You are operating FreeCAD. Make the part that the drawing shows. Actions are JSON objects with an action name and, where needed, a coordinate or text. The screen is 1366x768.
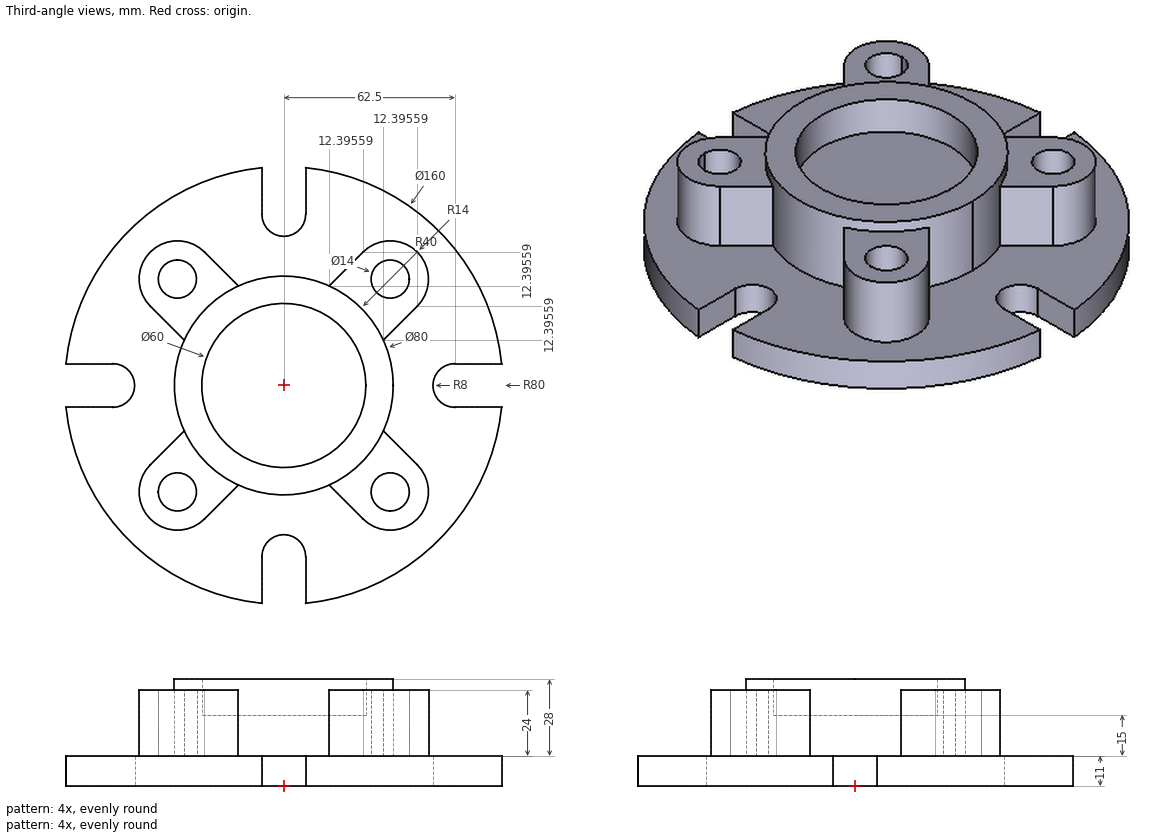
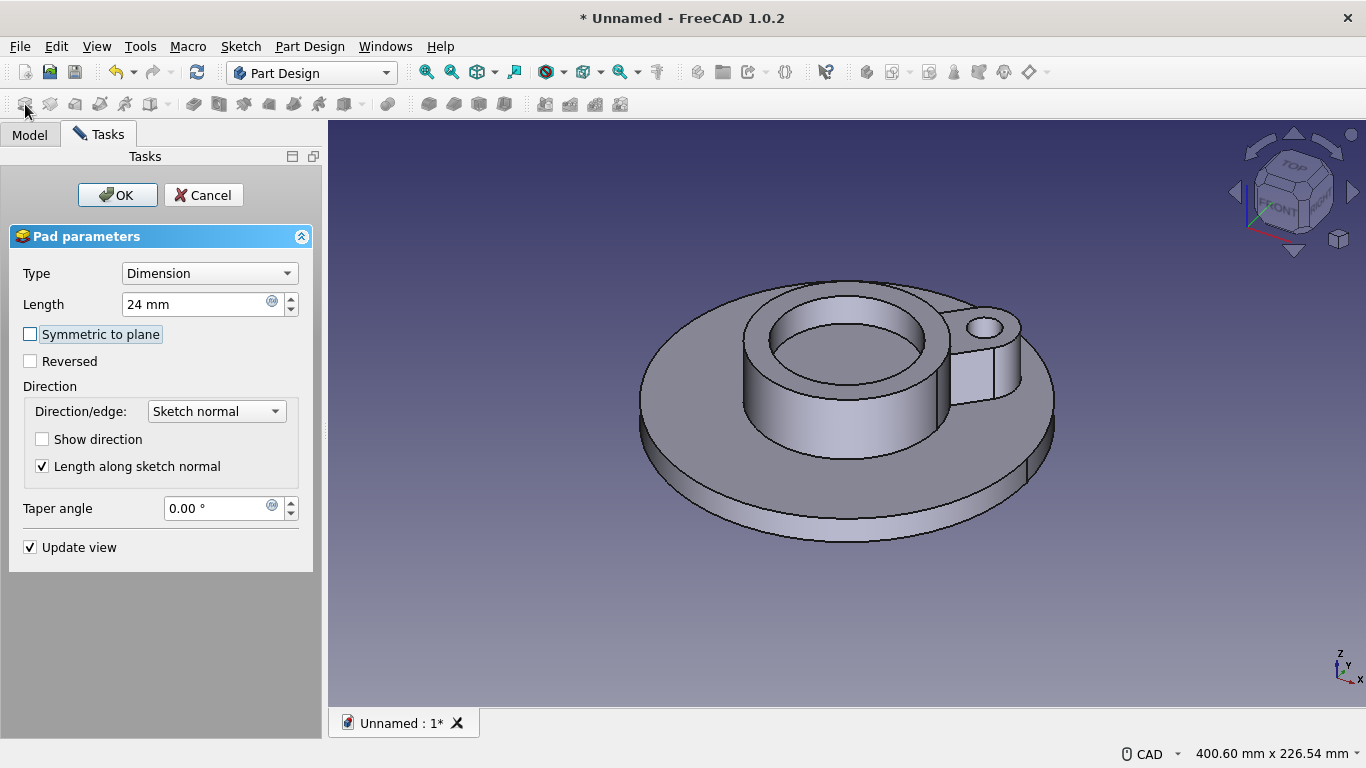
{"action": "left_click", "coordinate": [118, 195]}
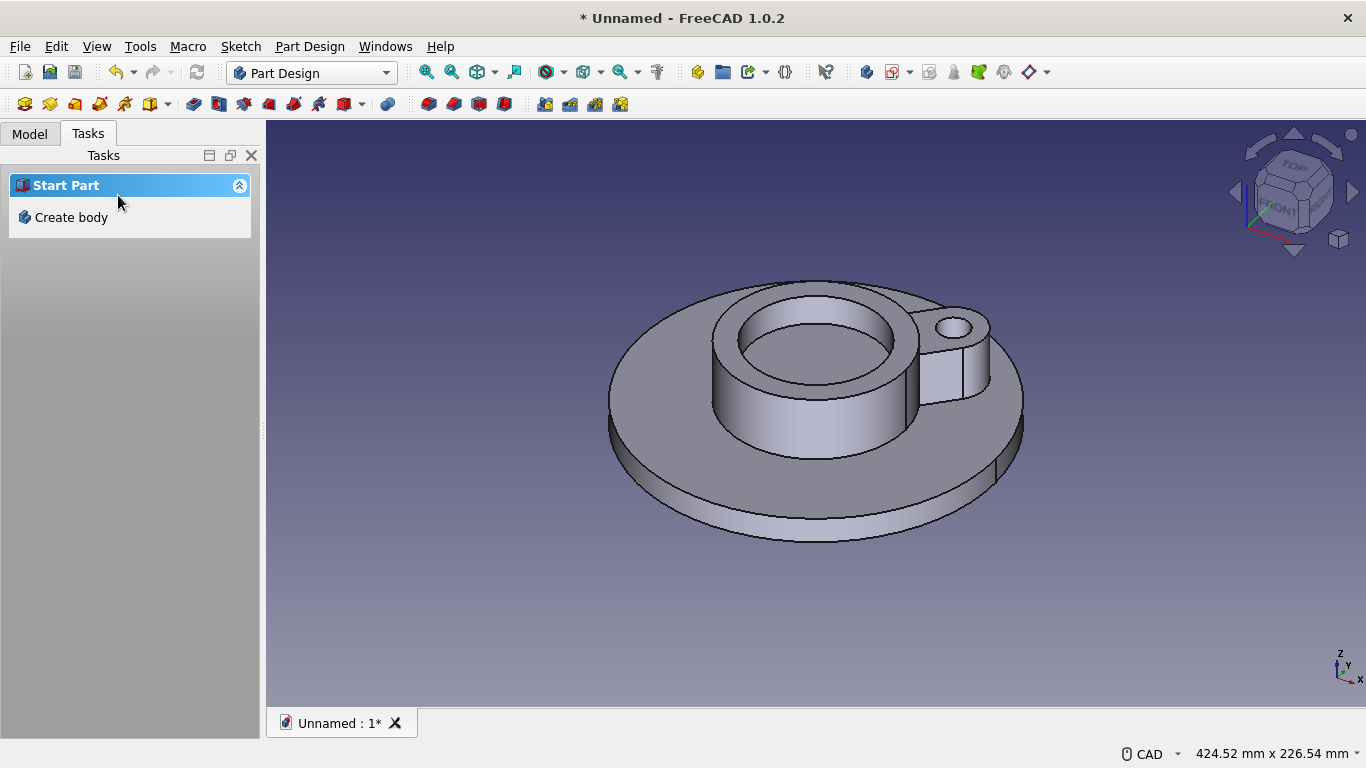
{"action": "left_click", "coordinate": [30, 134]}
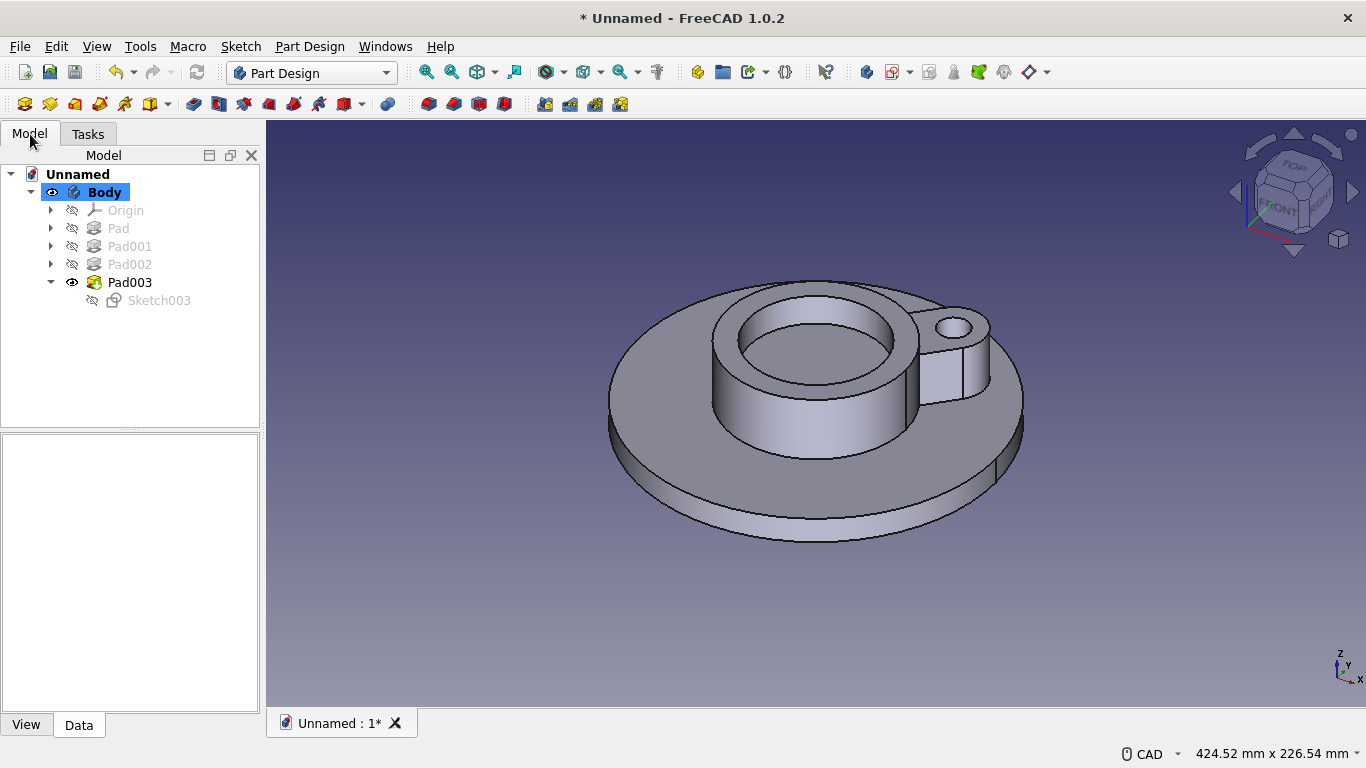
{"action": "left_click", "coordinate": [117, 282]}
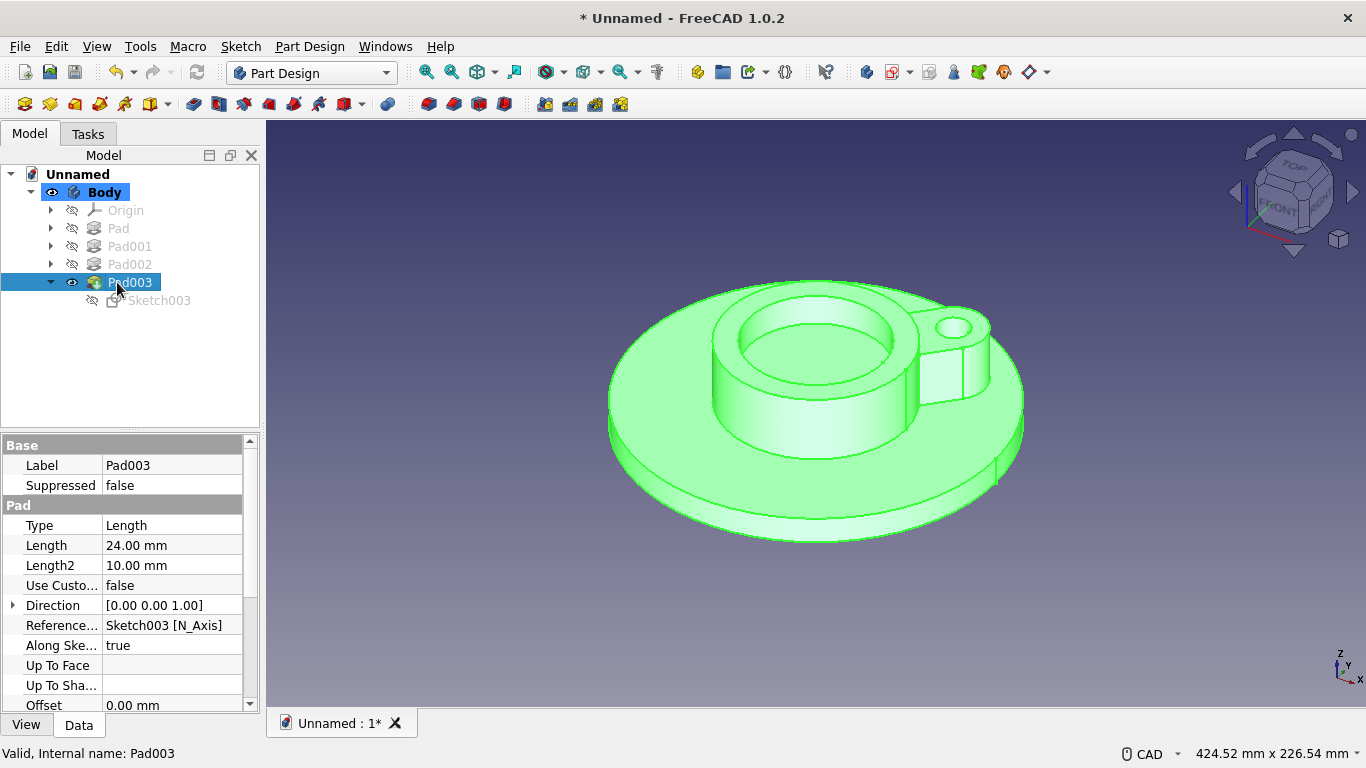
{"action": "left_click", "coordinate": [595, 104]}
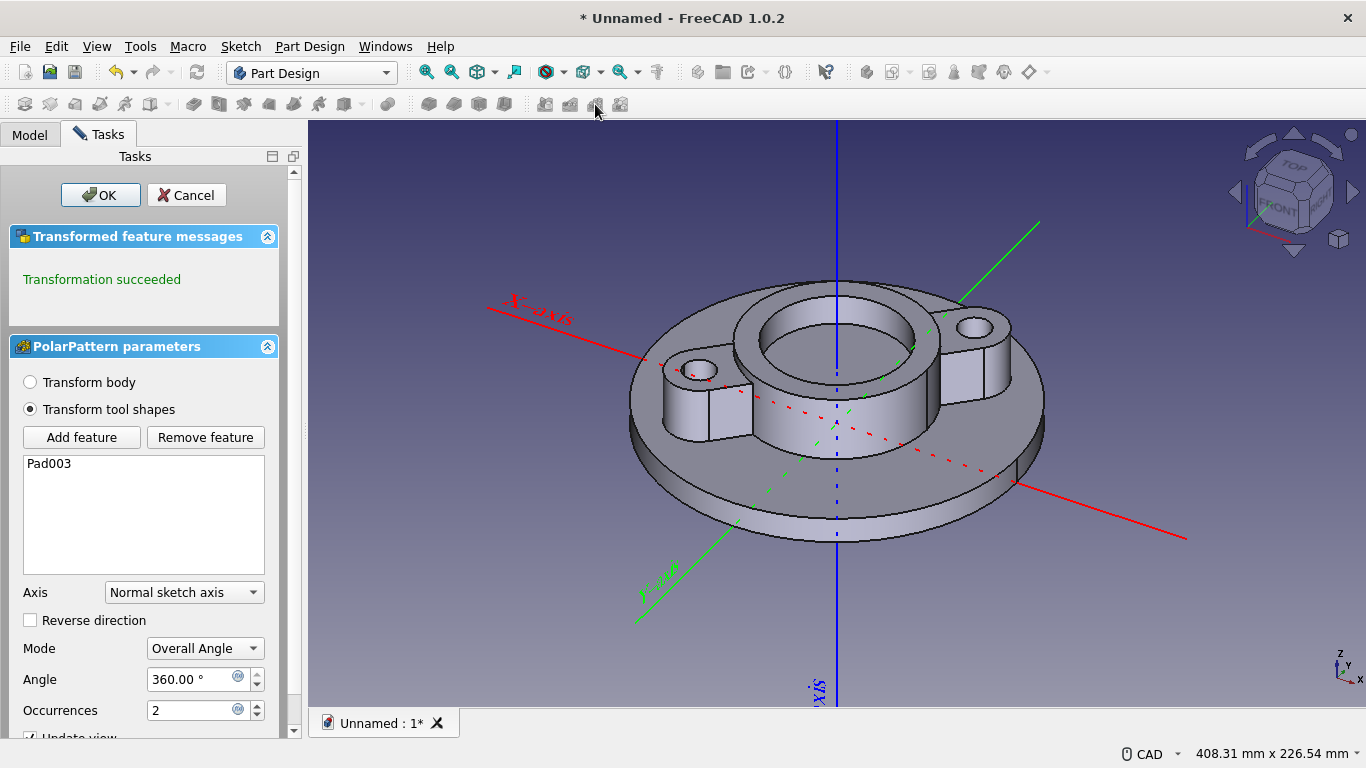
{"action": "left_click", "coordinate": [185, 592]}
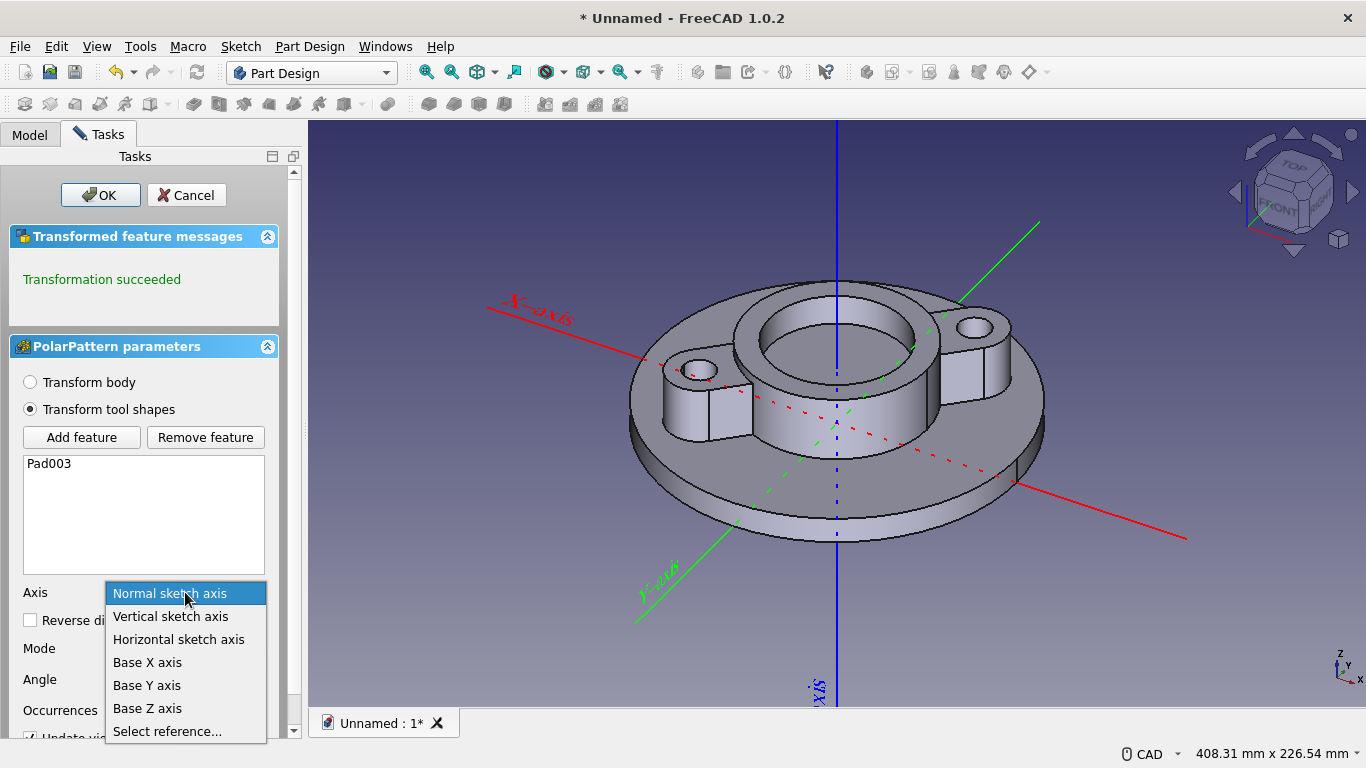
{"action": "left_click", "coordinate": [184, 708]}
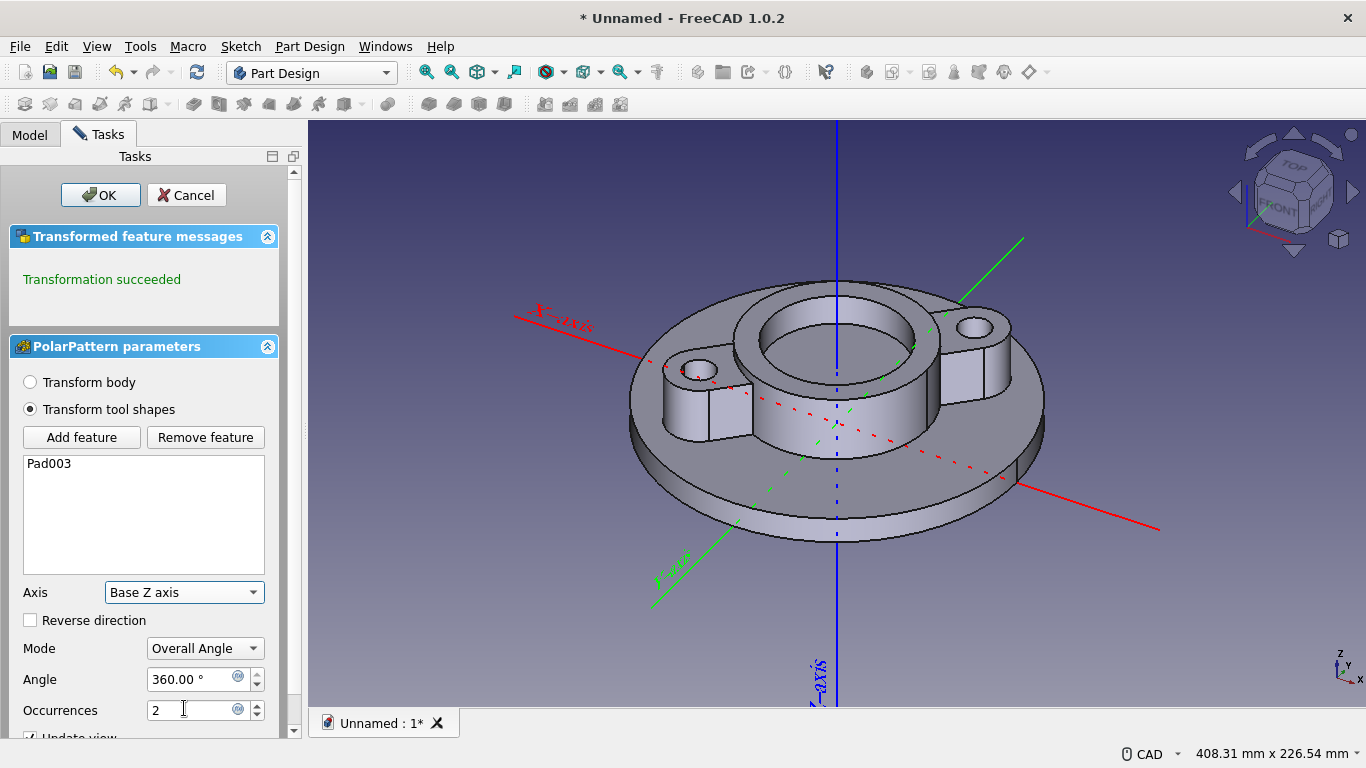
{"action": "triple_click", "coordinate": [199, 710]}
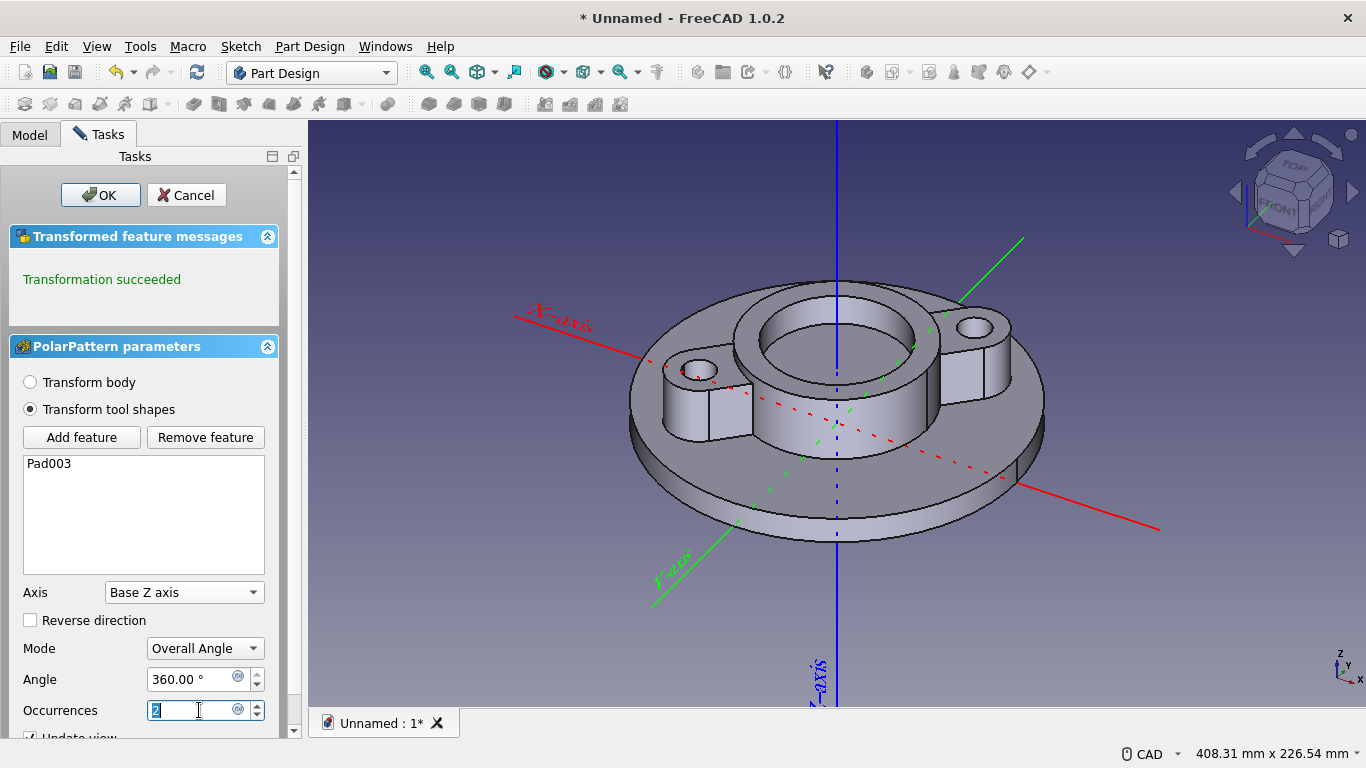
{"action": "type", "text": "4"}
{"action": "key", "text": "Tab"}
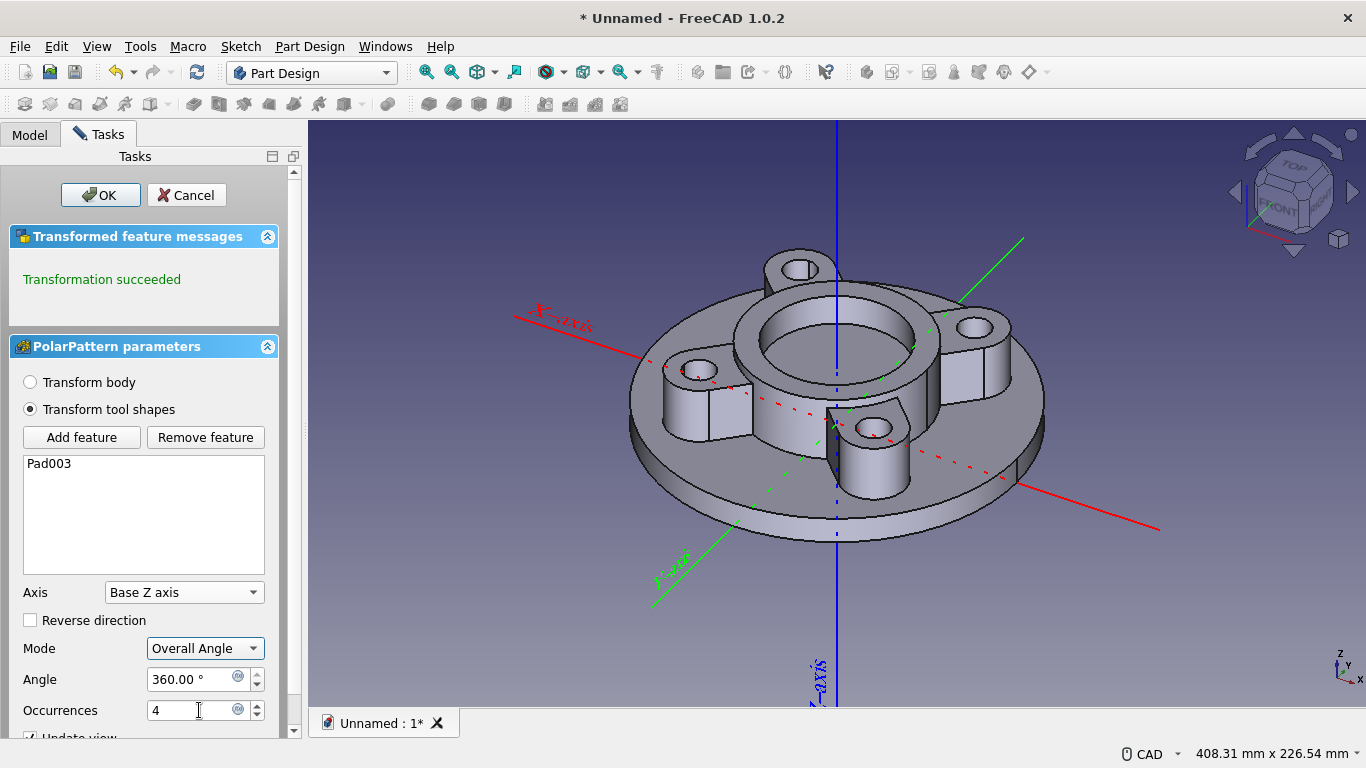
{"action": "left_click", "coordinate": [101, 195]}